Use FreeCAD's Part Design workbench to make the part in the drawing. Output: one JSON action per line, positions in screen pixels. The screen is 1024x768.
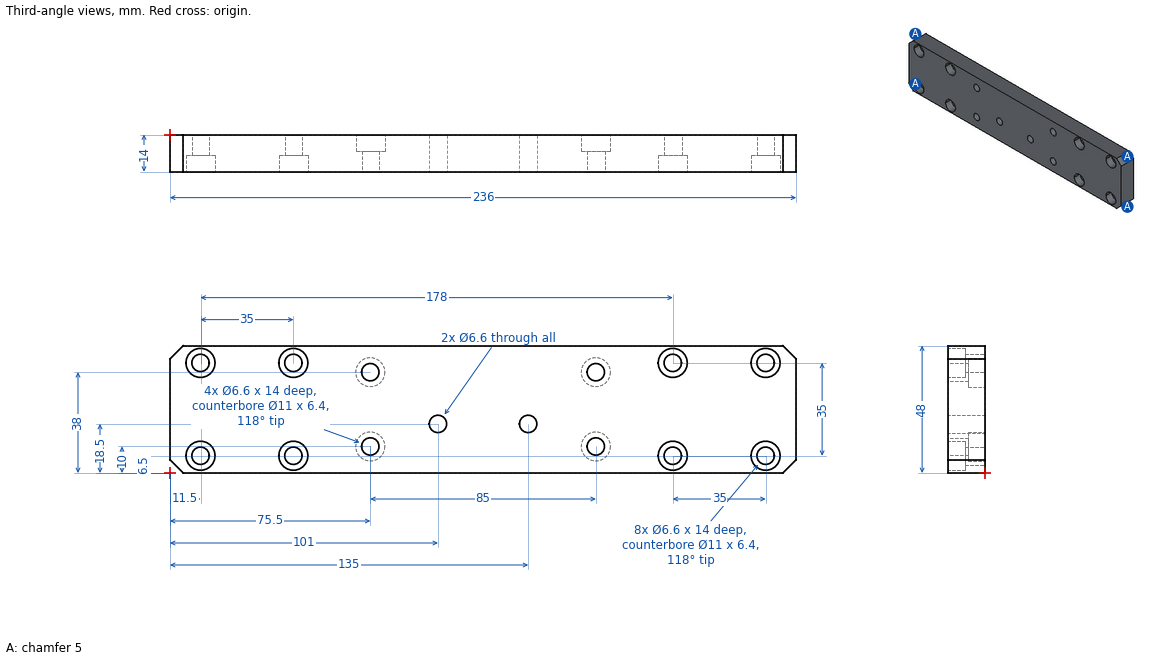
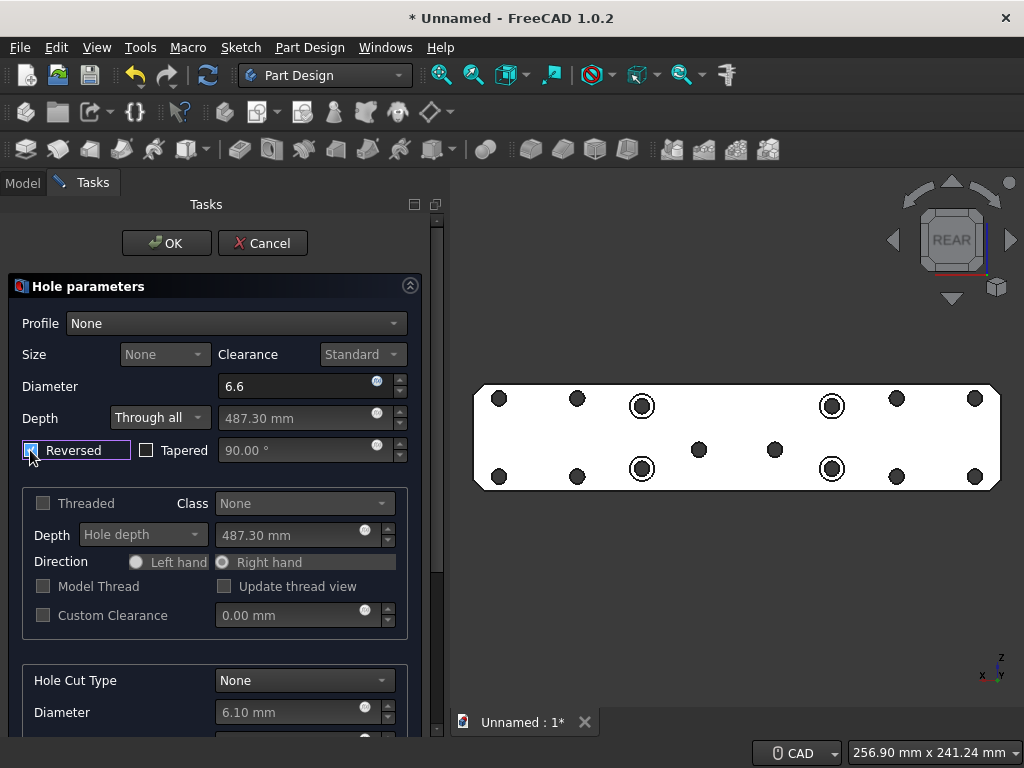
{"action": "left_click", "coordinate": [167, 243]}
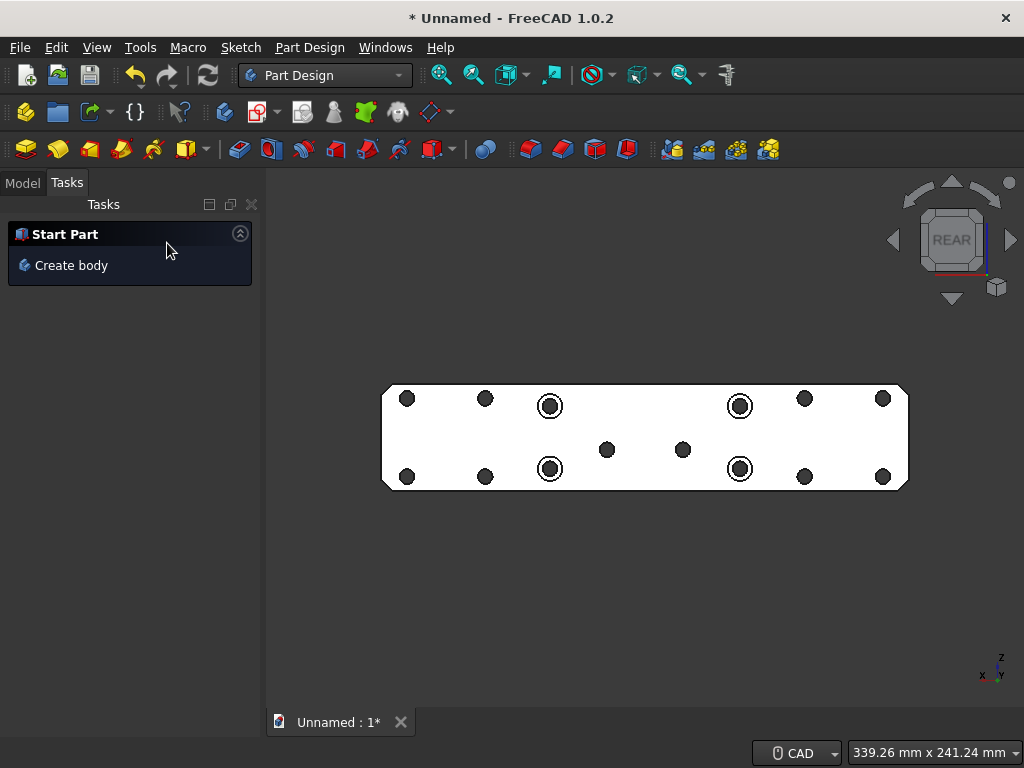
{"action": "key", "text": "0"}